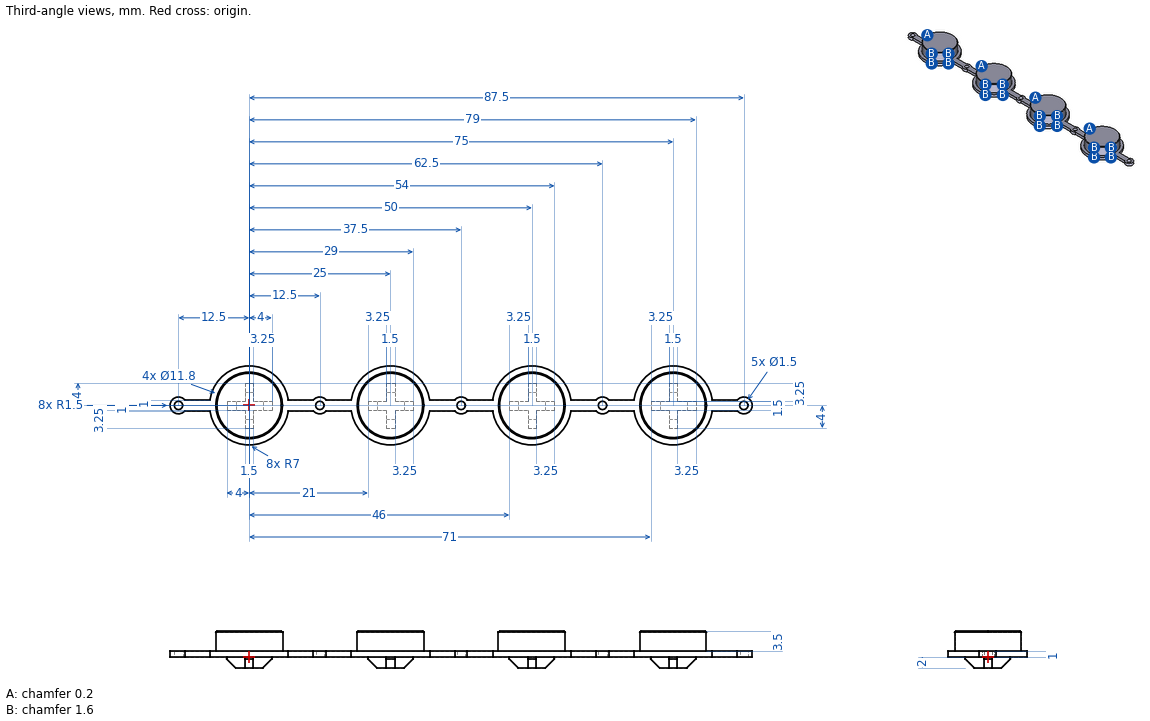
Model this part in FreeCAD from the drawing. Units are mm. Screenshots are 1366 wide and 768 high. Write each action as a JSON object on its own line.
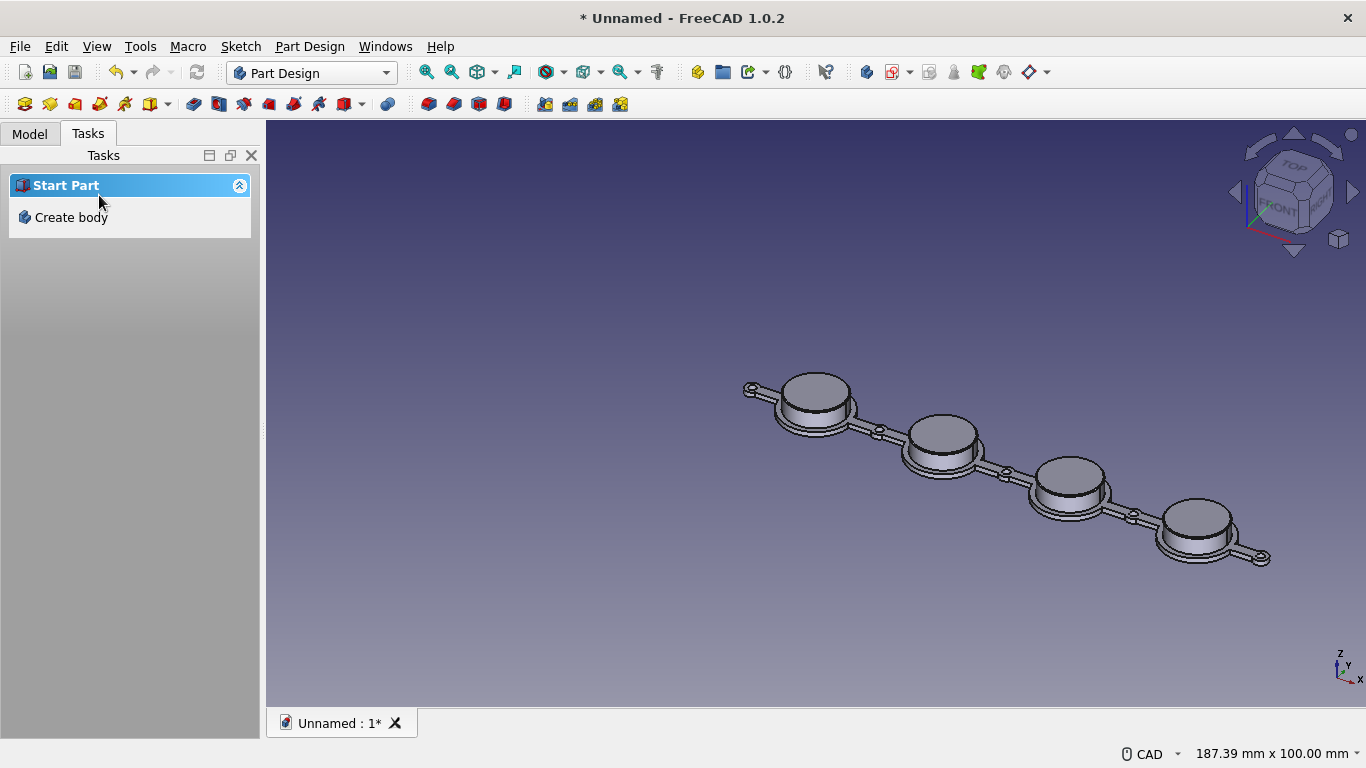
{"action": "left_click", "coordinate": [892, 72]}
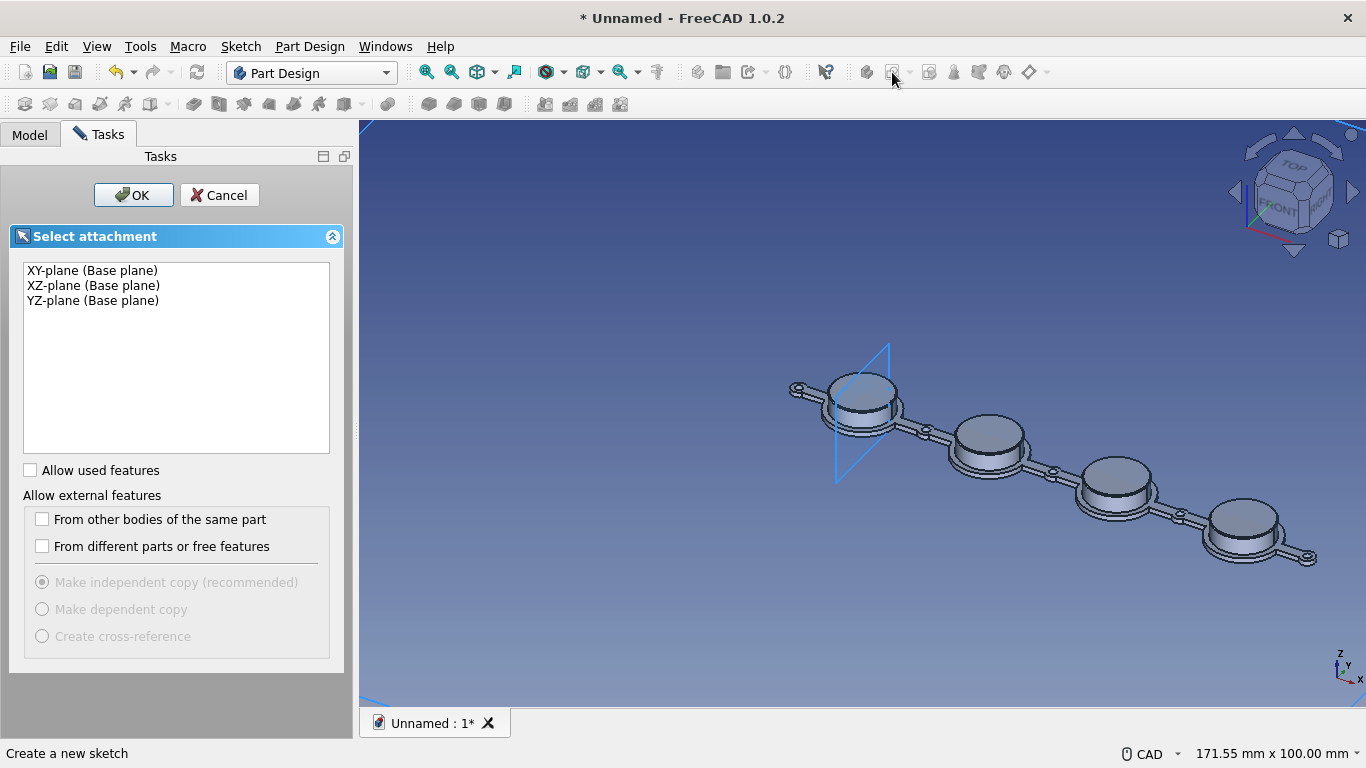
{"action": "left_click", "coordinate": [84, 270]}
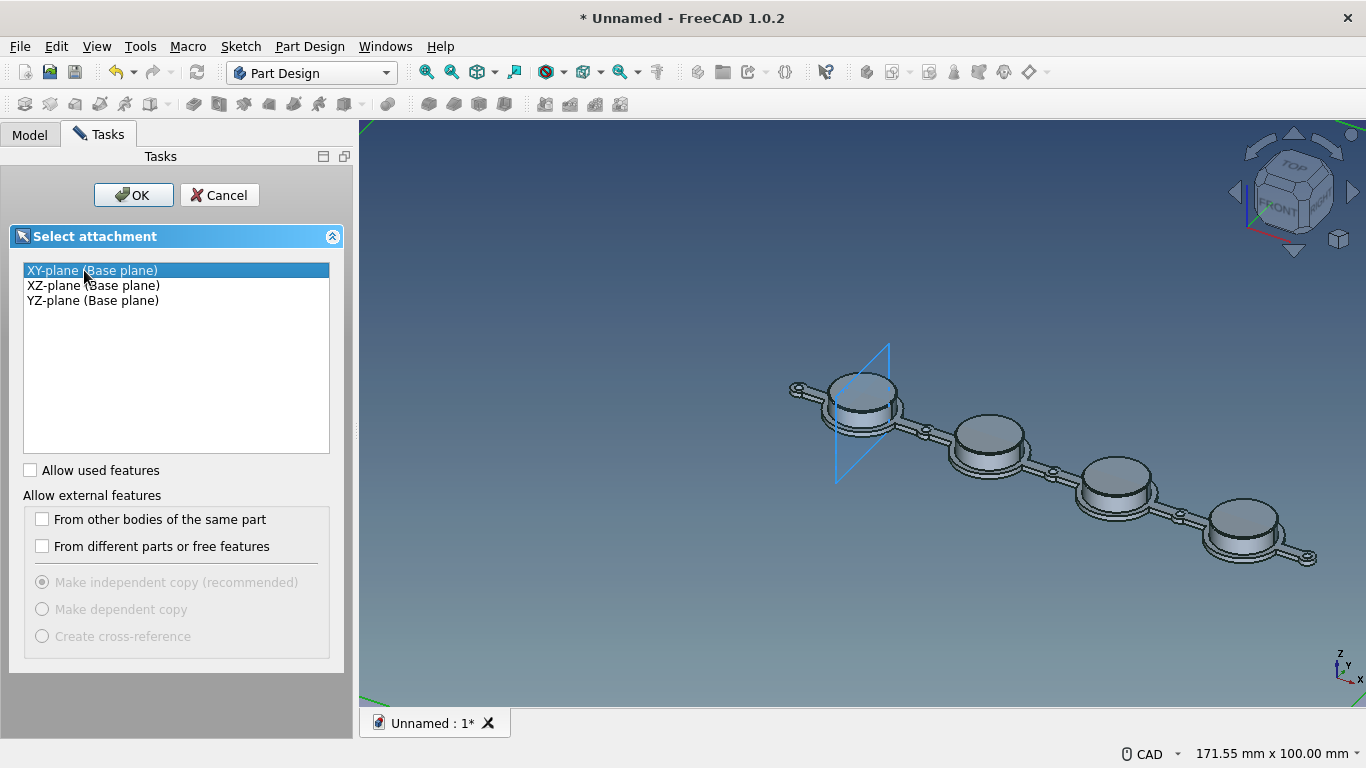
{"action": "left_click", "coordinate": [134, 195]}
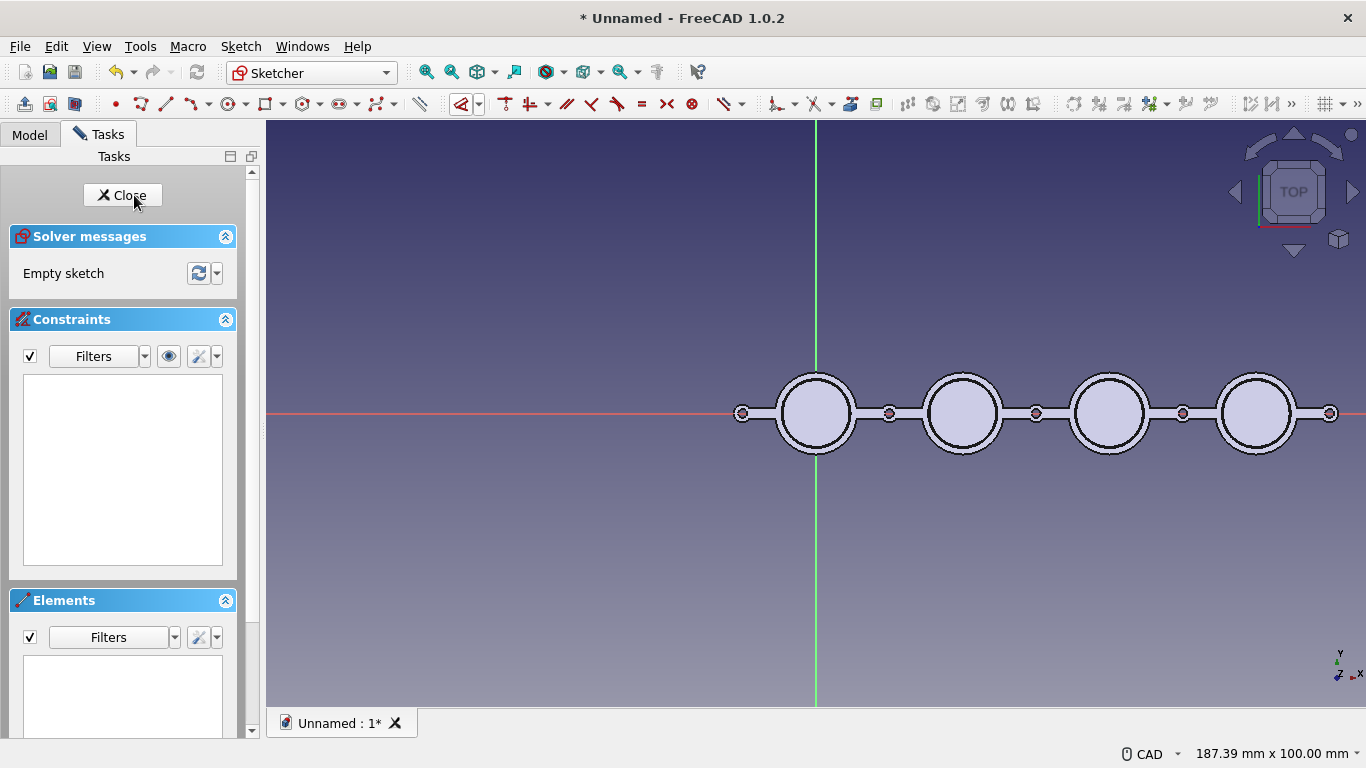
{"action": "key", "text": "q s"}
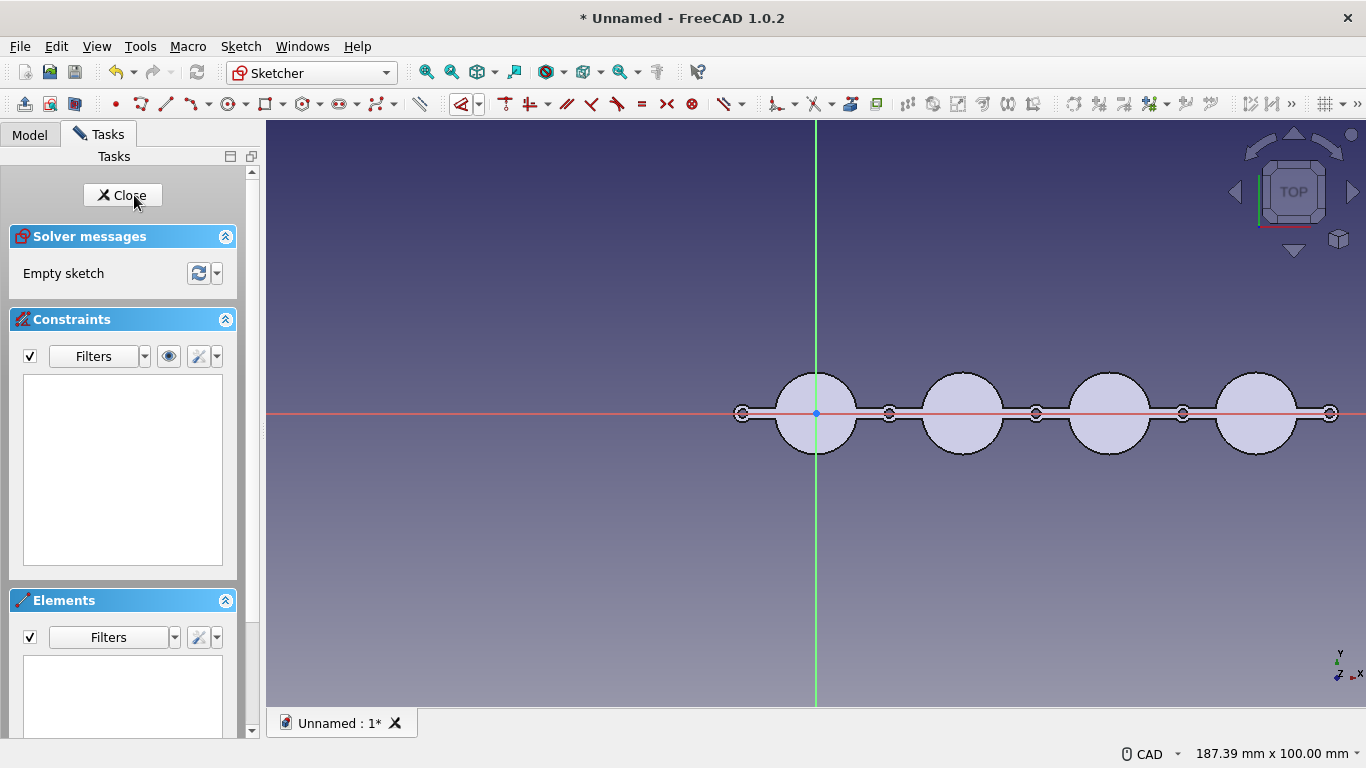
{"action": "scroll", "coordinate": [294, 413], "scroll_direction": "down", "scroll_amount": 1}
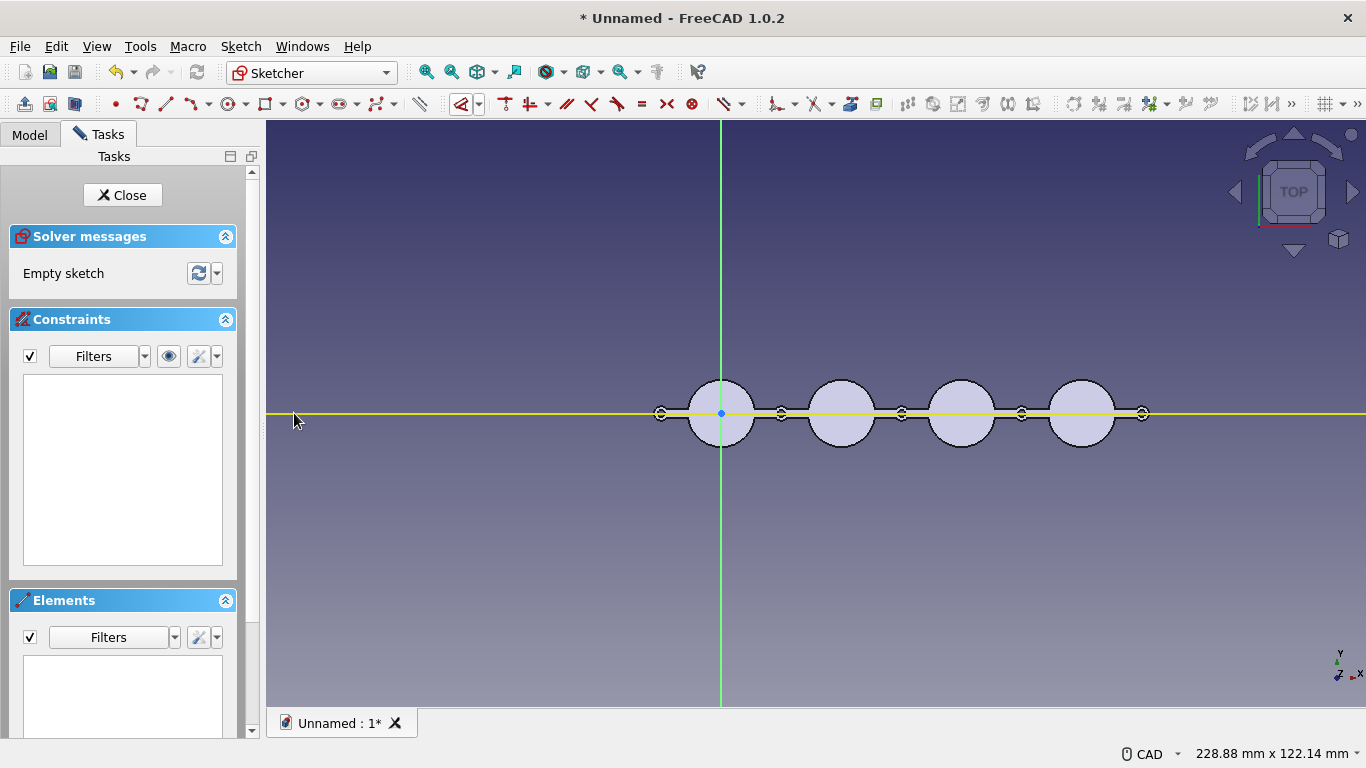
{"action": "scroll", "coordinate": [1201, 413], "scroll_direction": "up", "scroll_amount": 2}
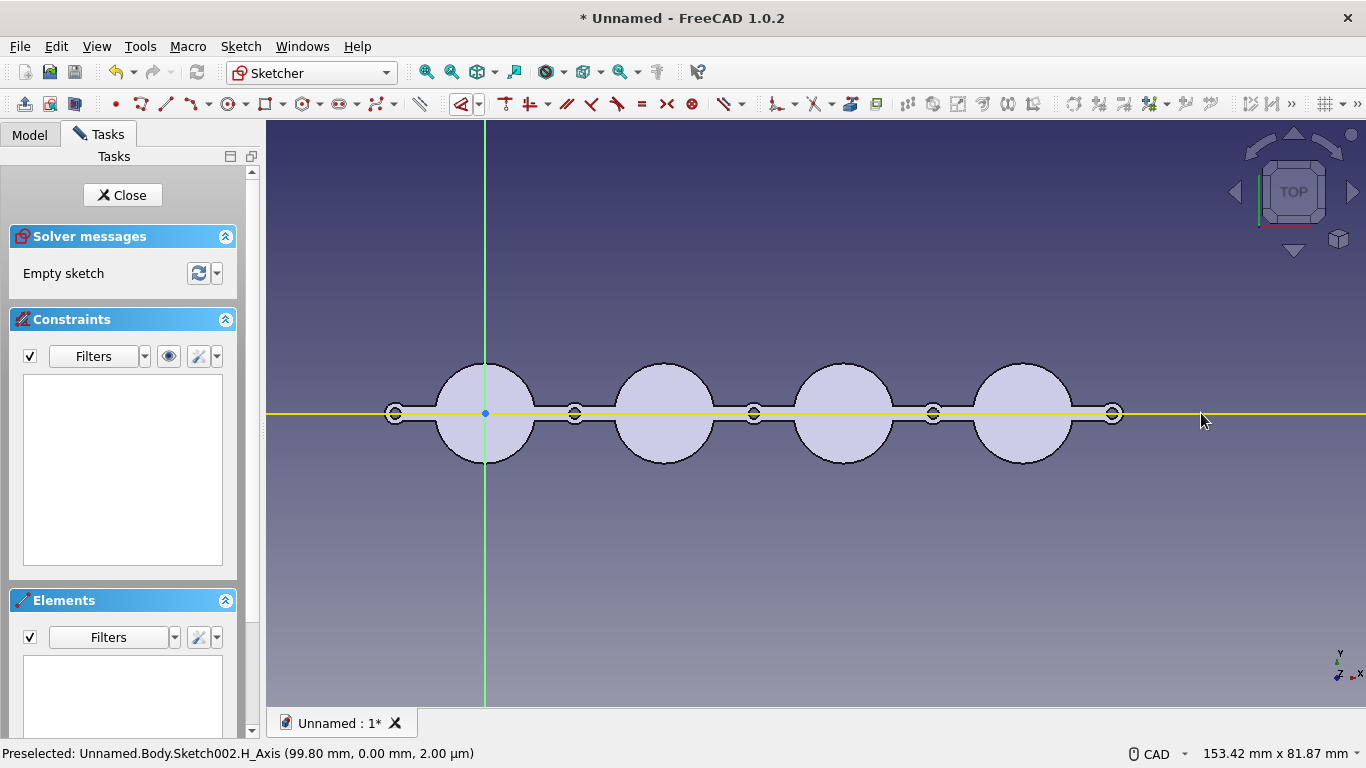
{"action": "key", "text": "g m"}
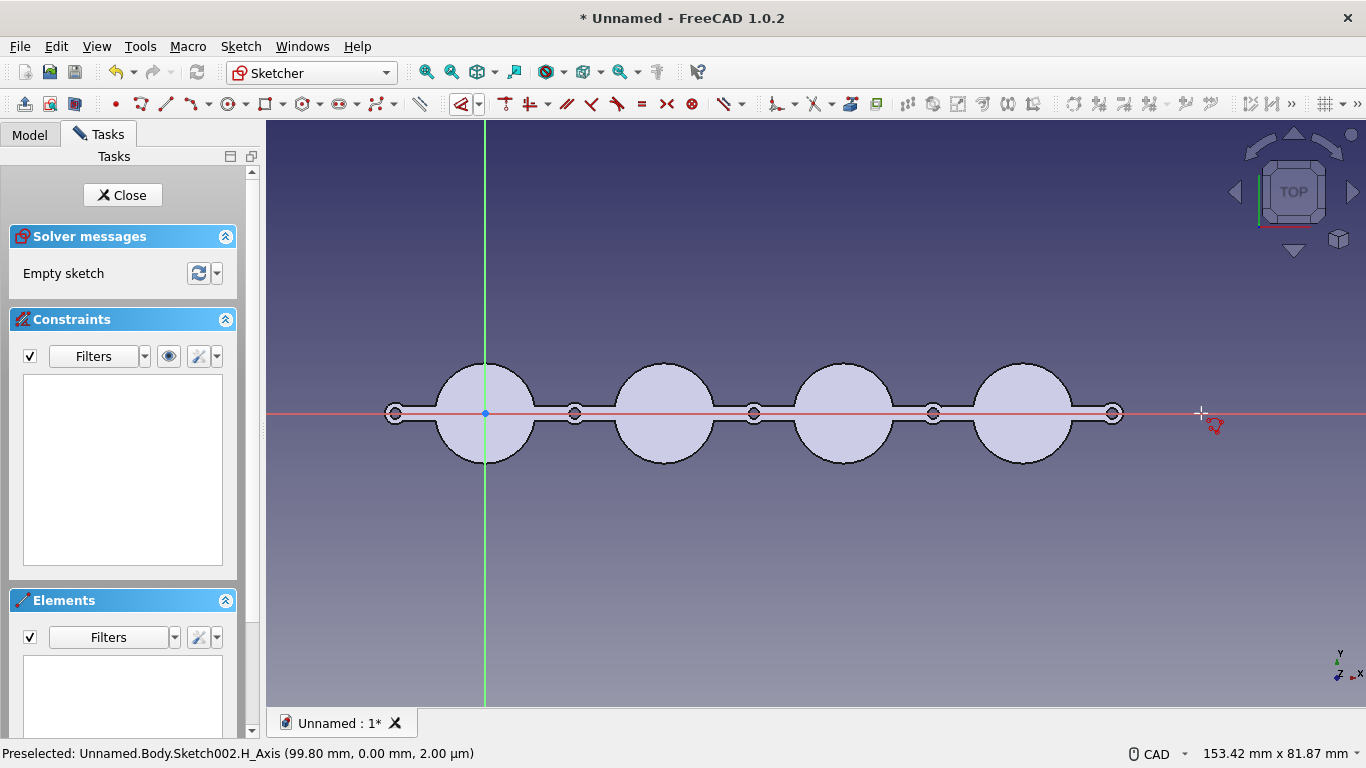
{"action": "scroll", "coordinate": [994, 419], "scroll_direction": "up", "scroll_amount": 6}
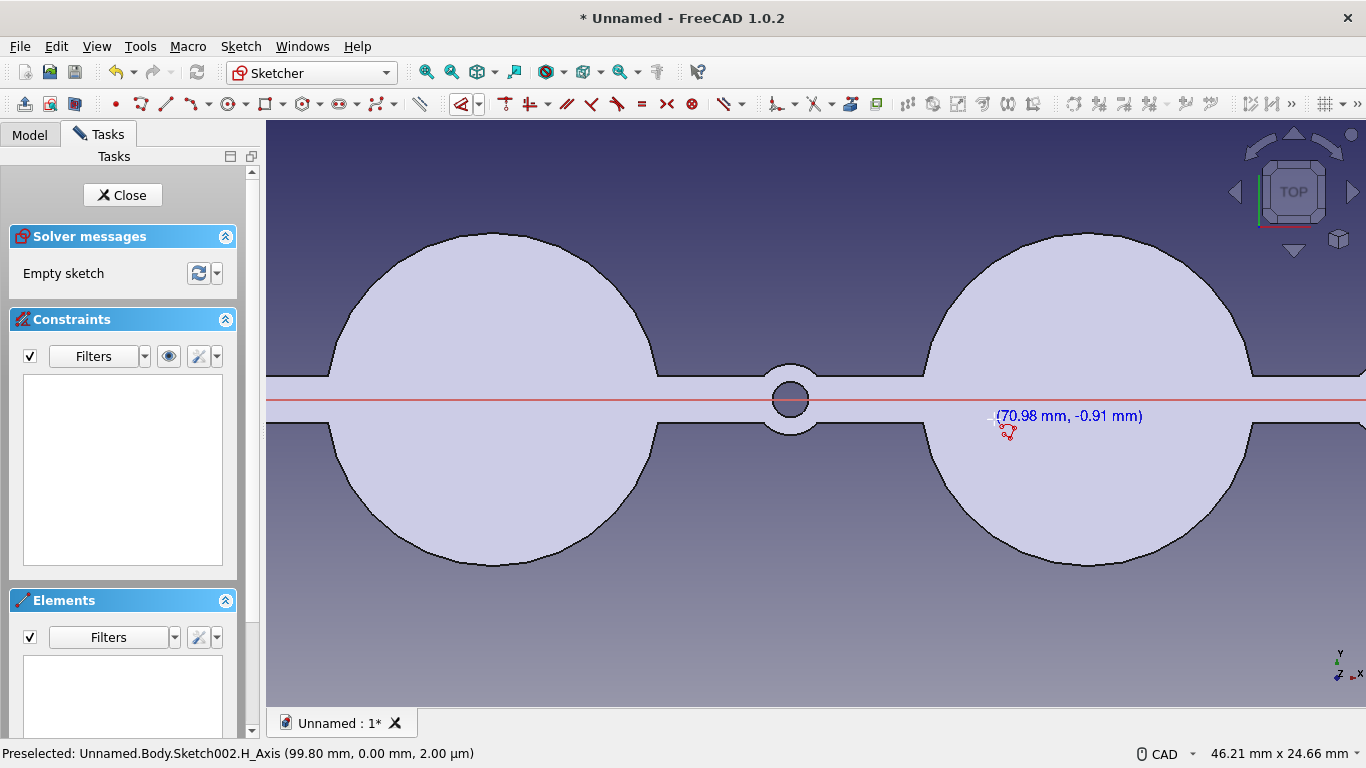
{"action": "left_click", "coordinate": [993, 417]}
{"action": "left_click", "coordinate": [993, 382]}
{"action": "left_click", "coordinate": [1070, 382]}
{"action": "left_click", "coordinate": [1070, 304]}
{"action": "left_click", "coordinate": [1106, 304]}
{"action": "left_click", "coordinate": [1106, 382]}
{"action": "left_click", "coordinate": [1183, 382]}
{"action": "left_click", "coordinate": [1183, 417]}
{"action": "left_click", "coordinate": [1106, 417]}
{"action": "left_click", "coordinate": [1106, 495]}
{"action": "left_click", "coordinate": [1070, 495]}
{"action": "left_click", "coordinate": [1070, 417]}
{"action": "left_click", "coordinate": [993, 418]}